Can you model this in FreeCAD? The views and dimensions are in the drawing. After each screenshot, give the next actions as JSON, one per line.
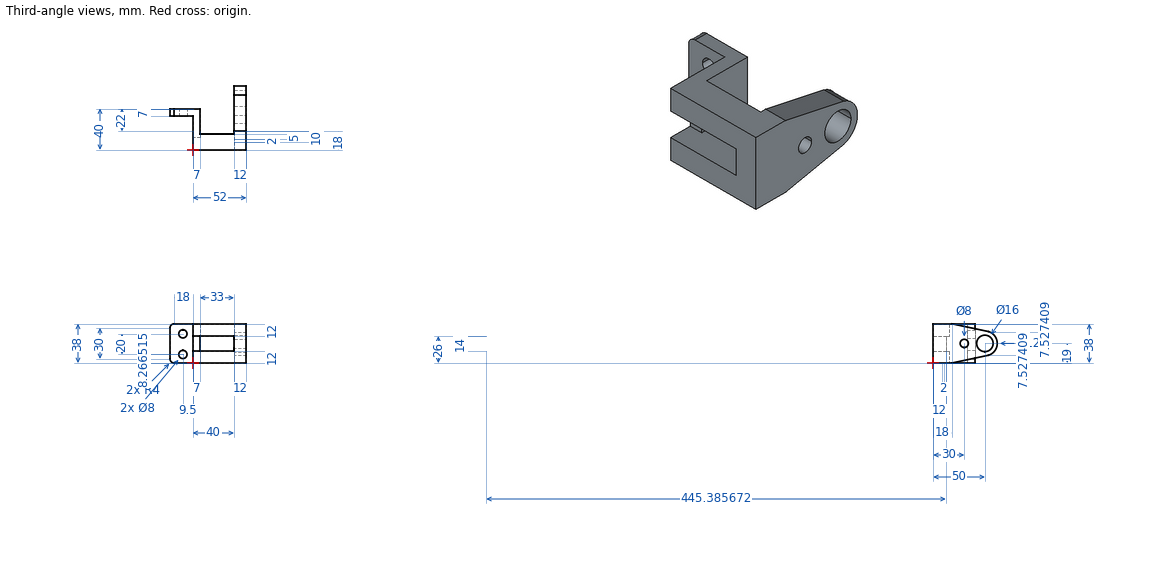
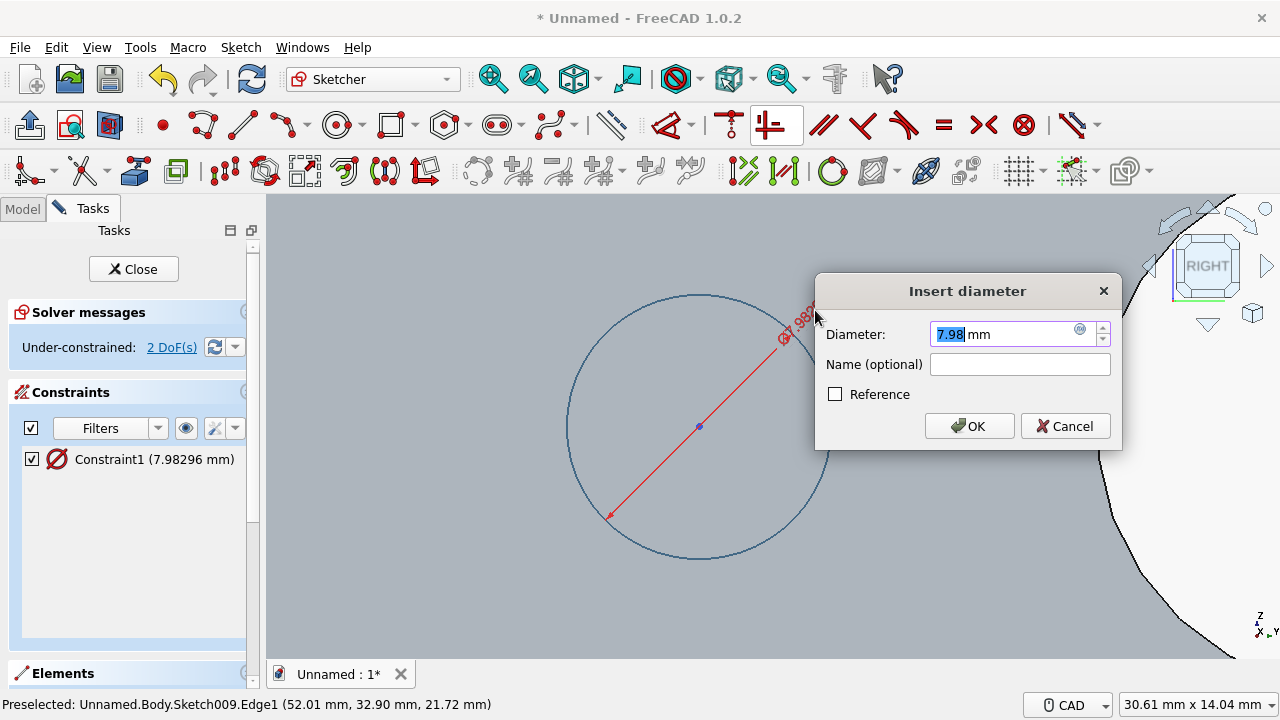
{"action": "type", "text": "8"}
{"action": "key", "text": "Return"}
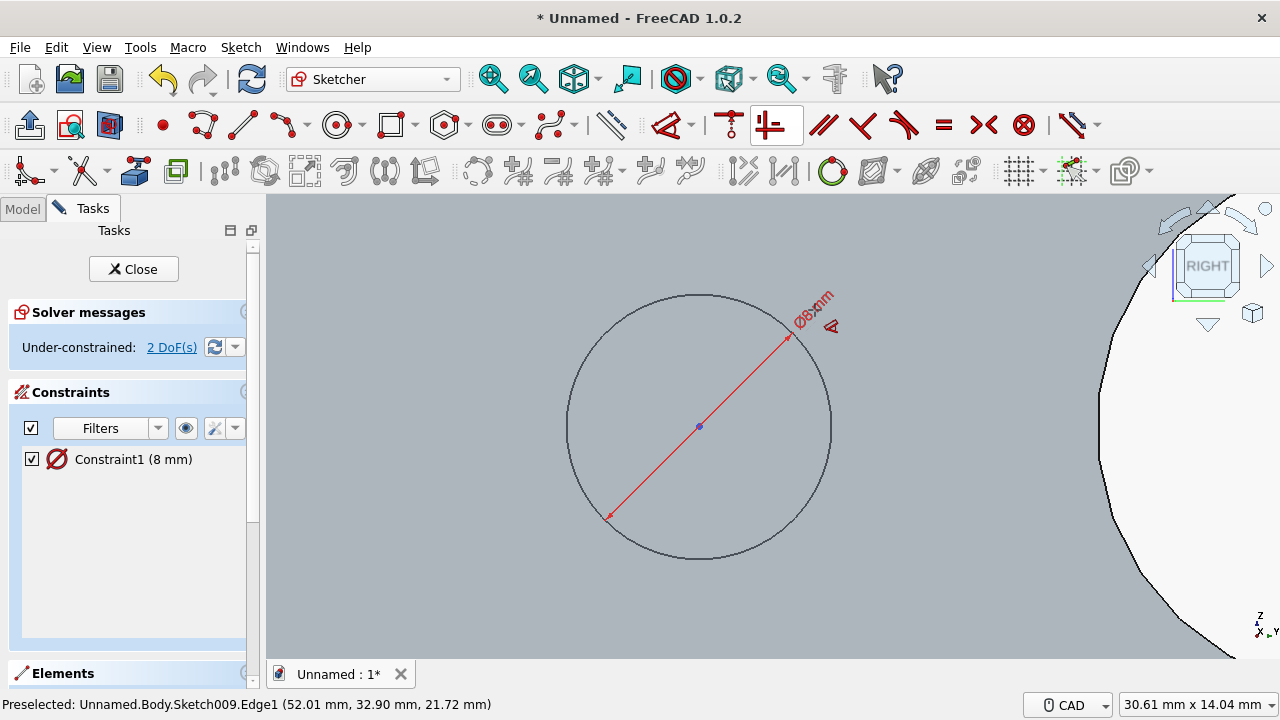
{"action": "left_click", "coordinate": [699, 427]}
{"action": "left_click", "coordinate": [497, 393]}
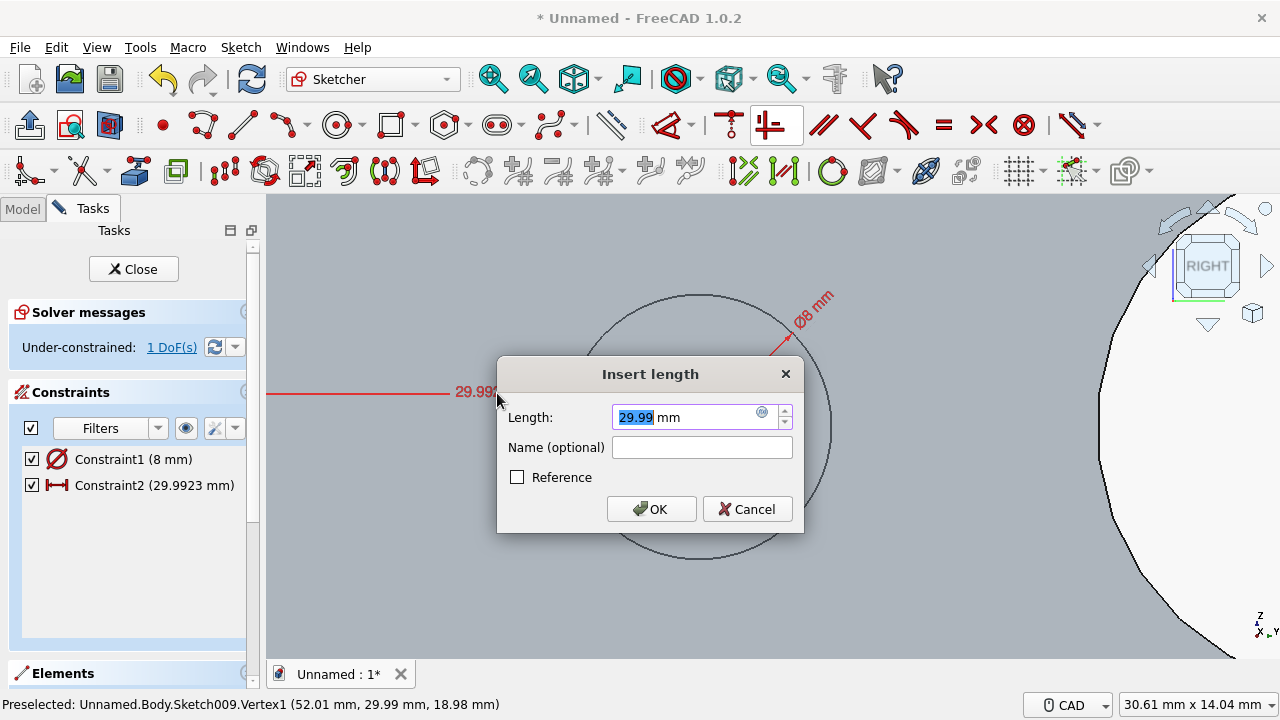
{"action": "type", "text": "30"}
{"action": "key", "text": "Return"}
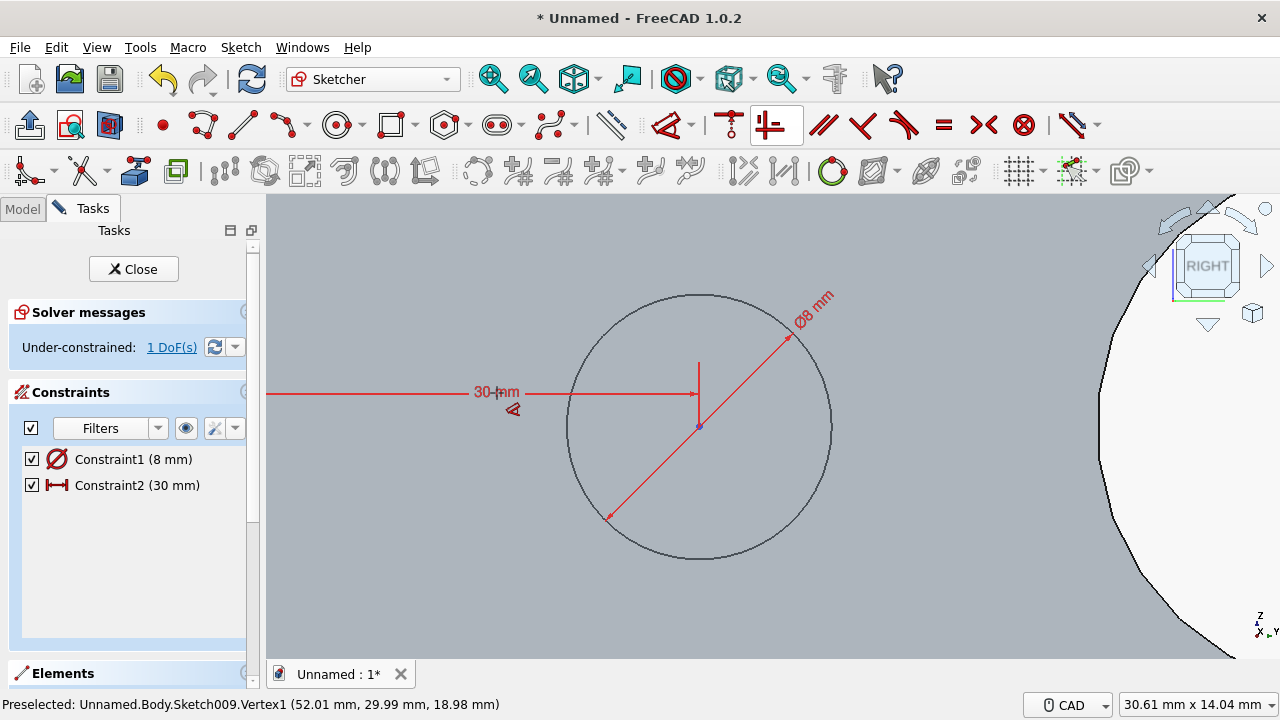
{"action": "left_click", "coordinate": [699, 427]}
{"action": "left_click", "coordinate": [733, 529]}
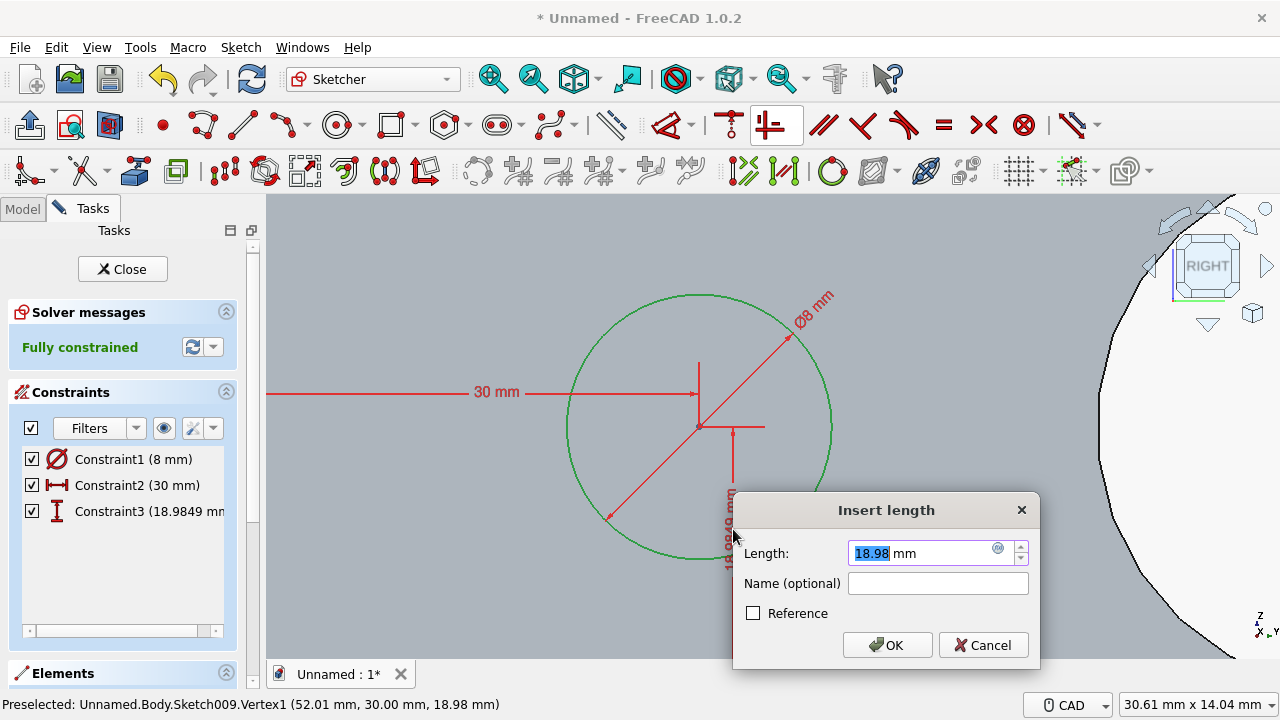
{"action": "type", "text": "19"}
{"action": "key", "text": "Return"}
{"action": "key", "text": "Escape"}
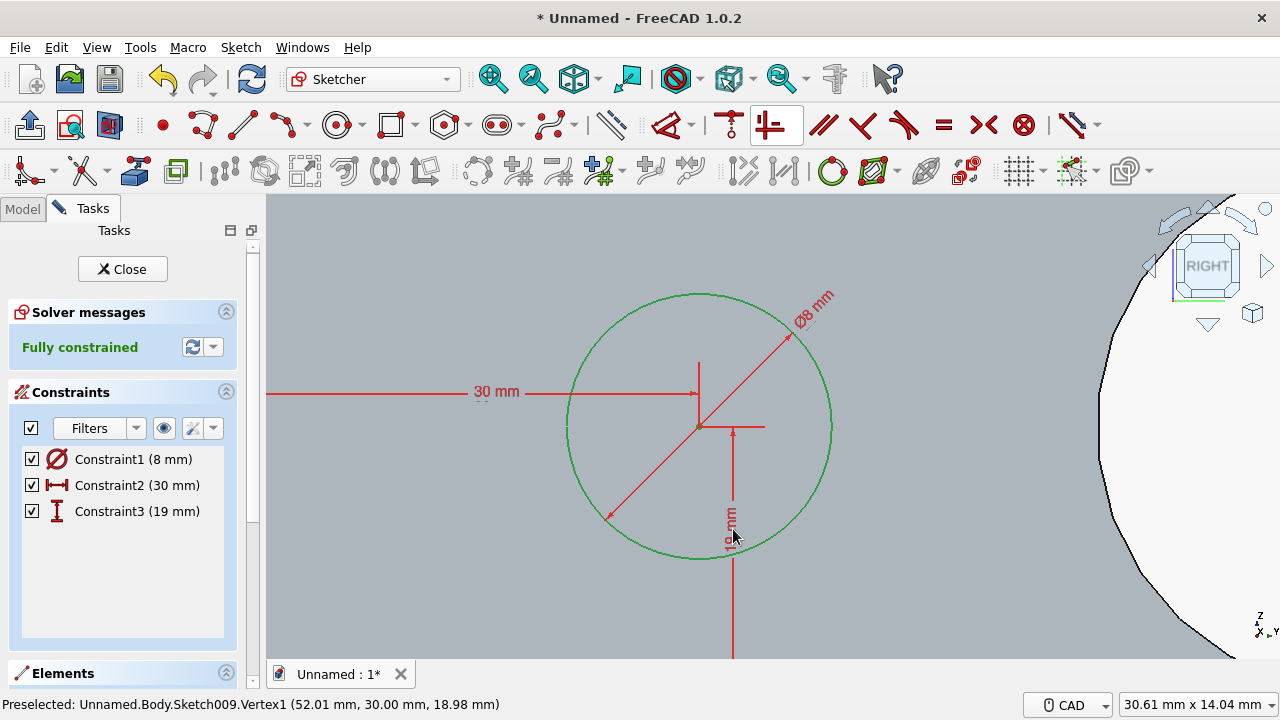
{"action": "left_click", "coordinate": [123, 269]}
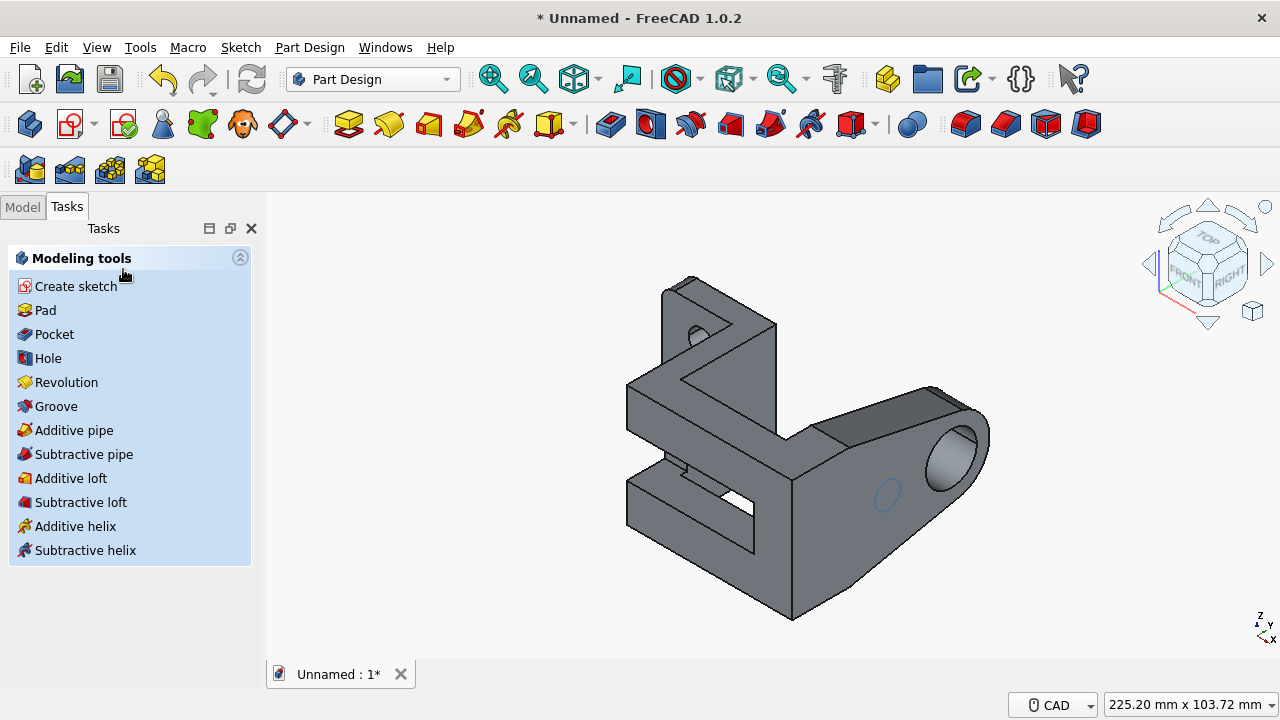
{"action": "left_click", "coordinate": [612, 124]}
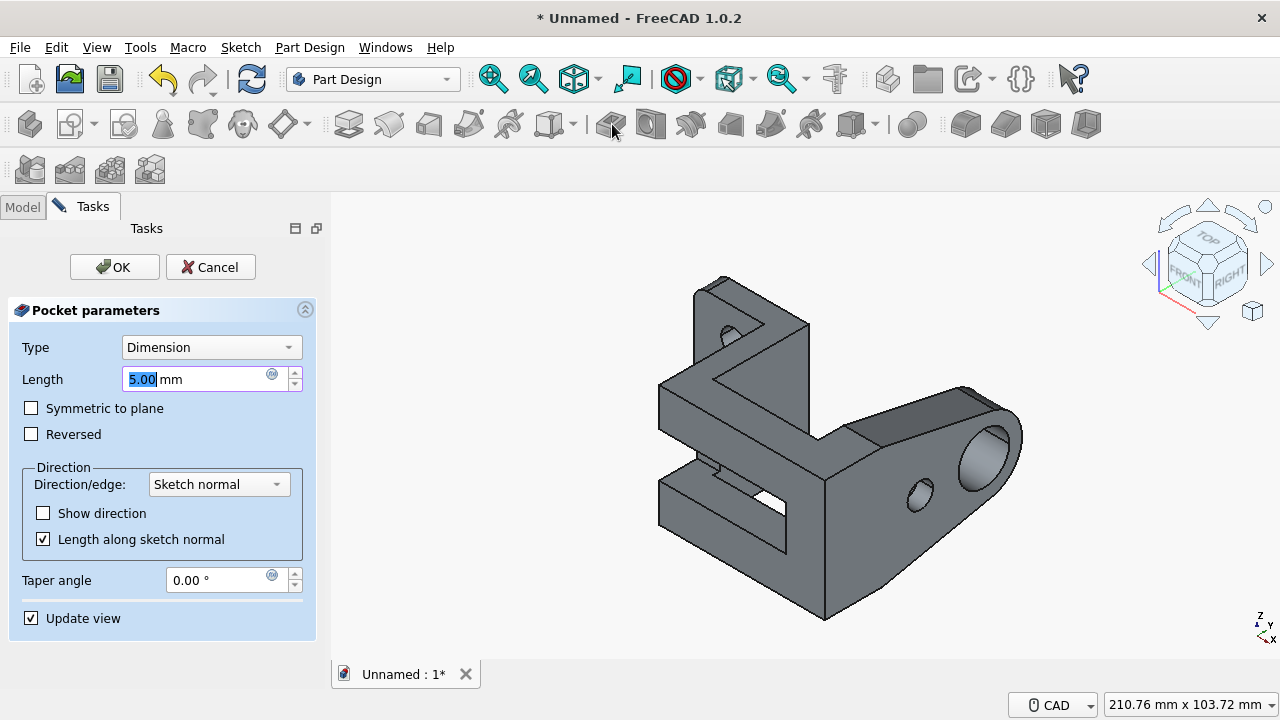
{"action": "type", "text": "12"}
{"action": "key", "text": "Tab"}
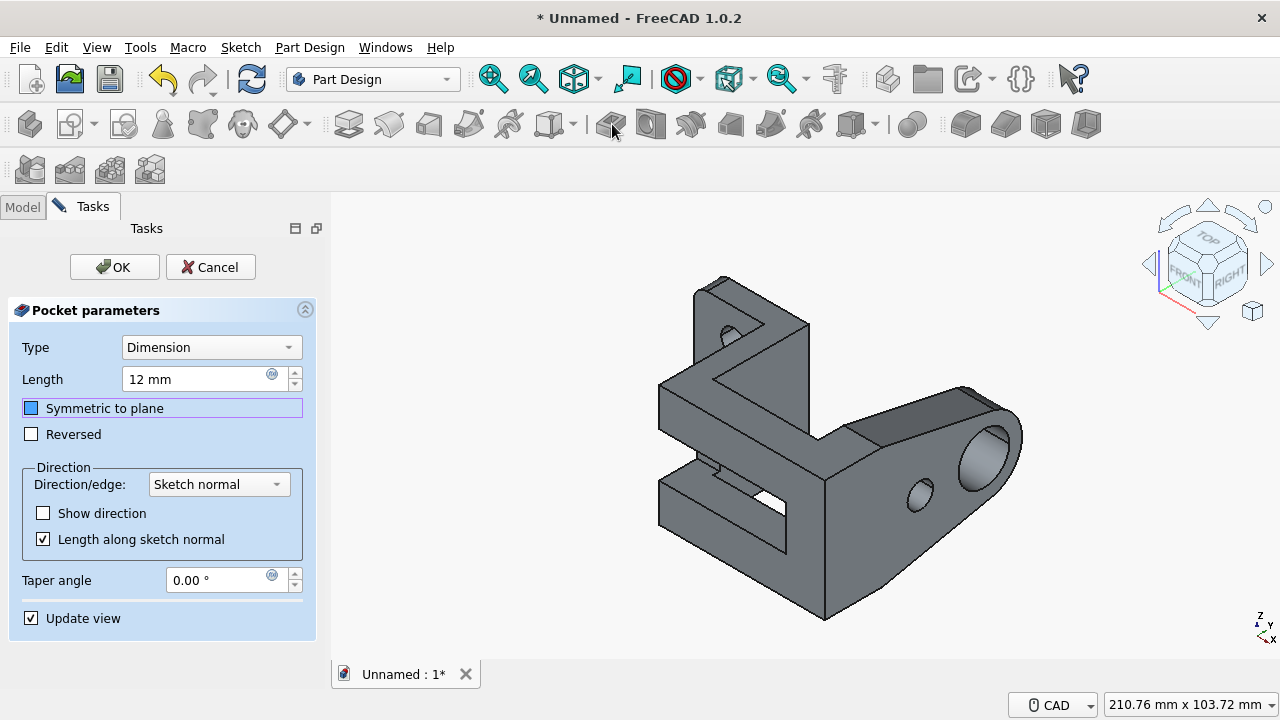
{"action": "left_click", "coordinate": [115, 267]}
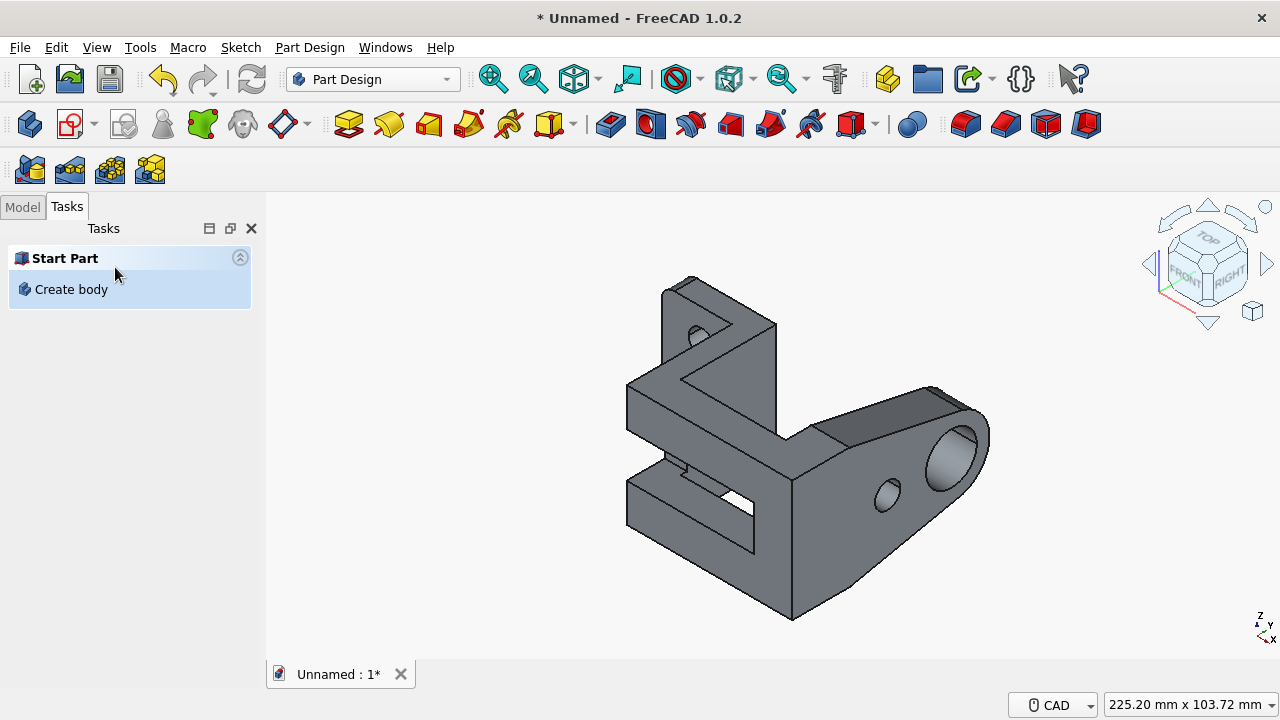
{"action": "key", "text": "4"}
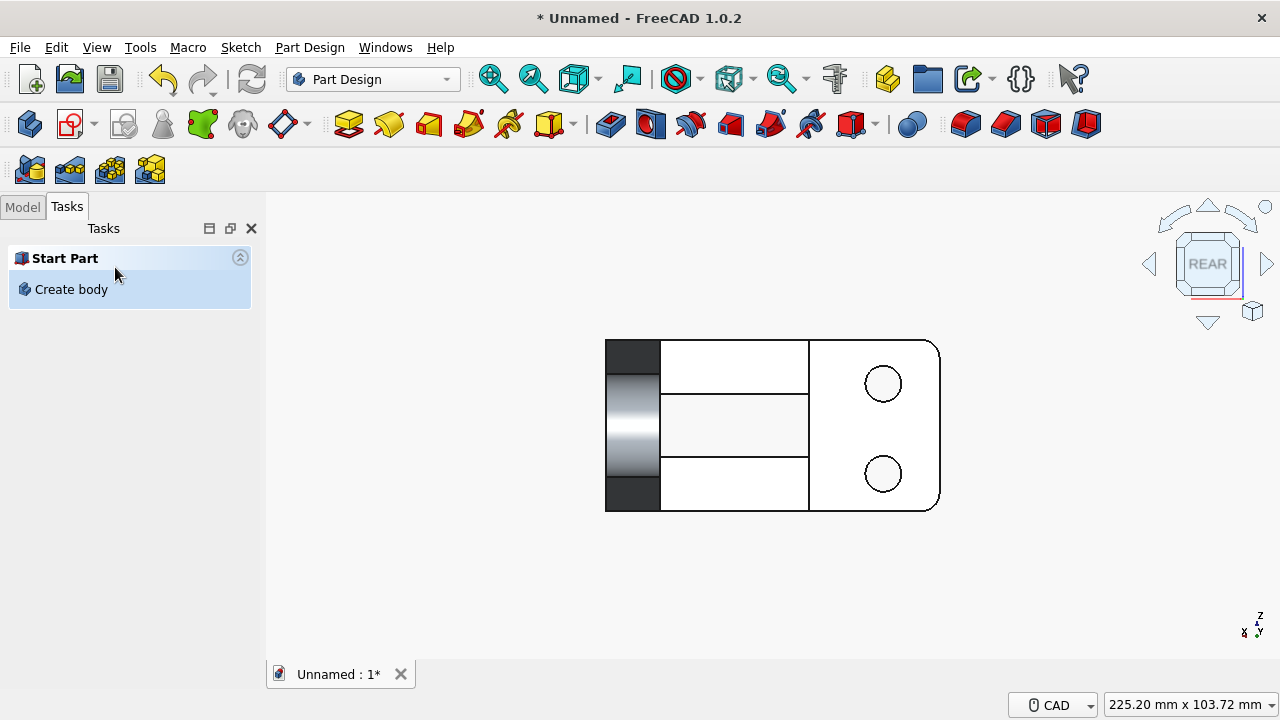
{"action": "left_click", "coordinate": [494, 80]}